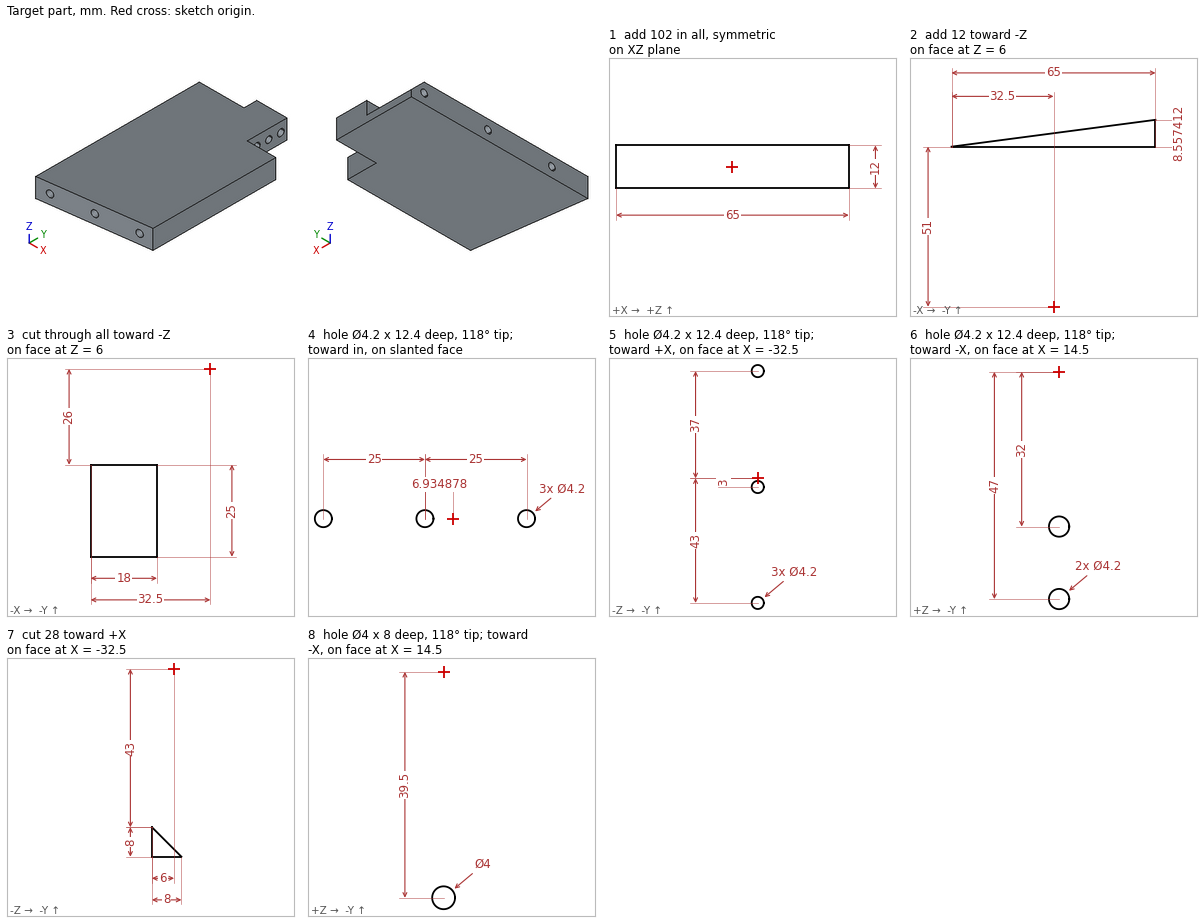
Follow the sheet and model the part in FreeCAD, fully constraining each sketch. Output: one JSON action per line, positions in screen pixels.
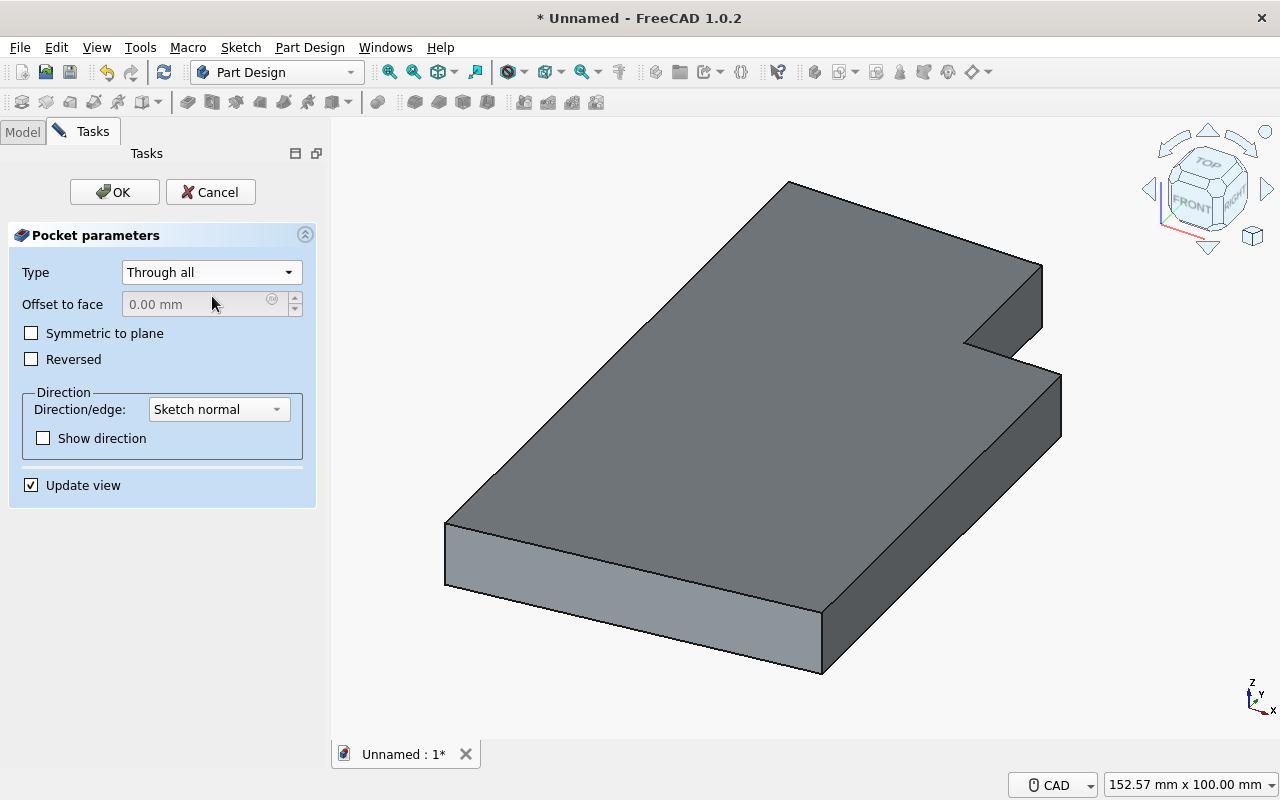
{"action": "left_click", "coordinate": [115, 192]}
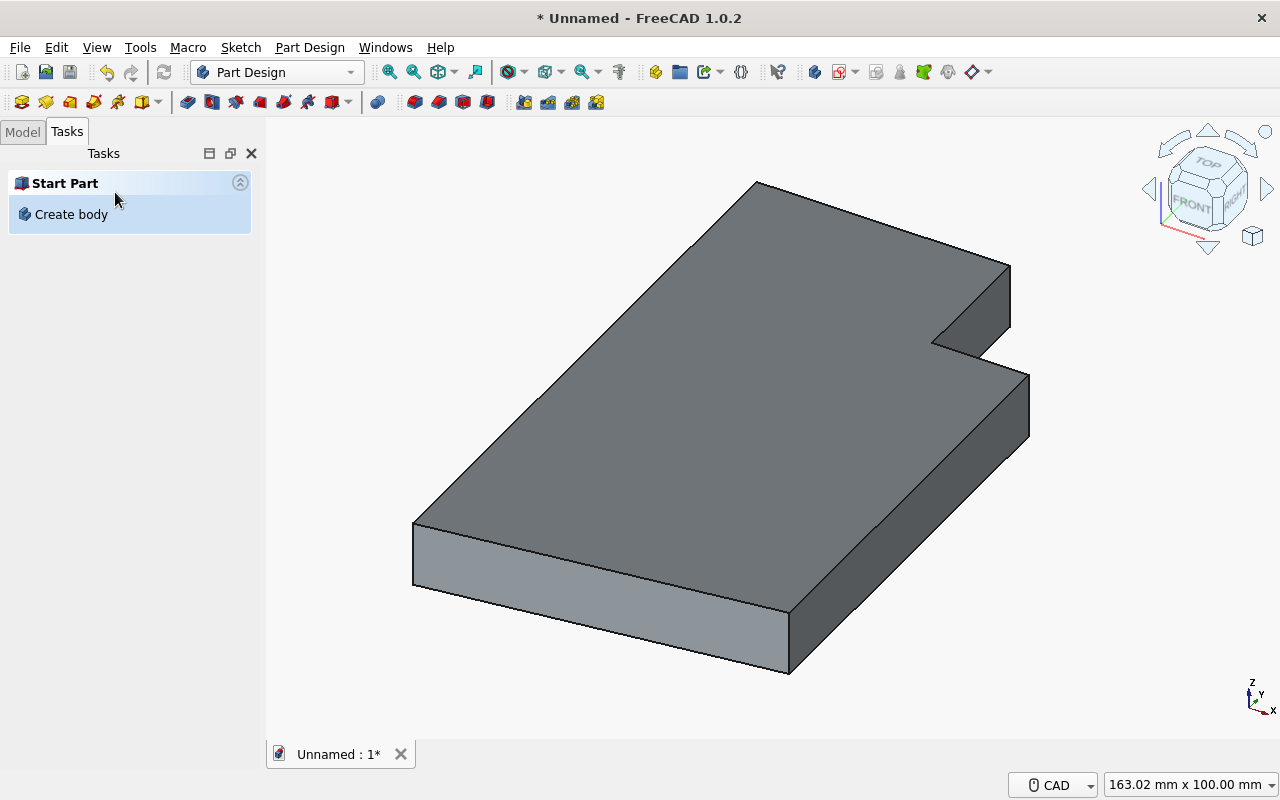
{"action": "left_click", "coordinate": [709, 623]}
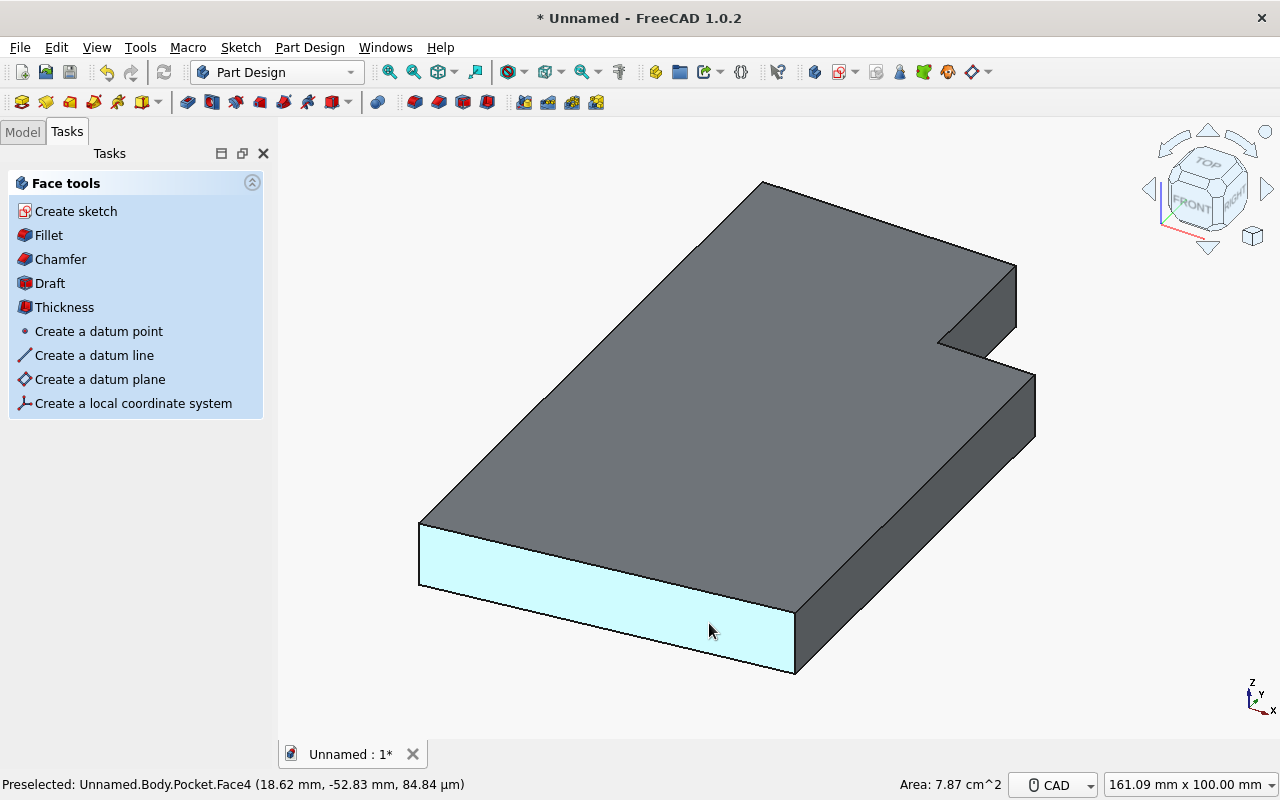
{"action": "left_click", "coordinate": [840, 72]}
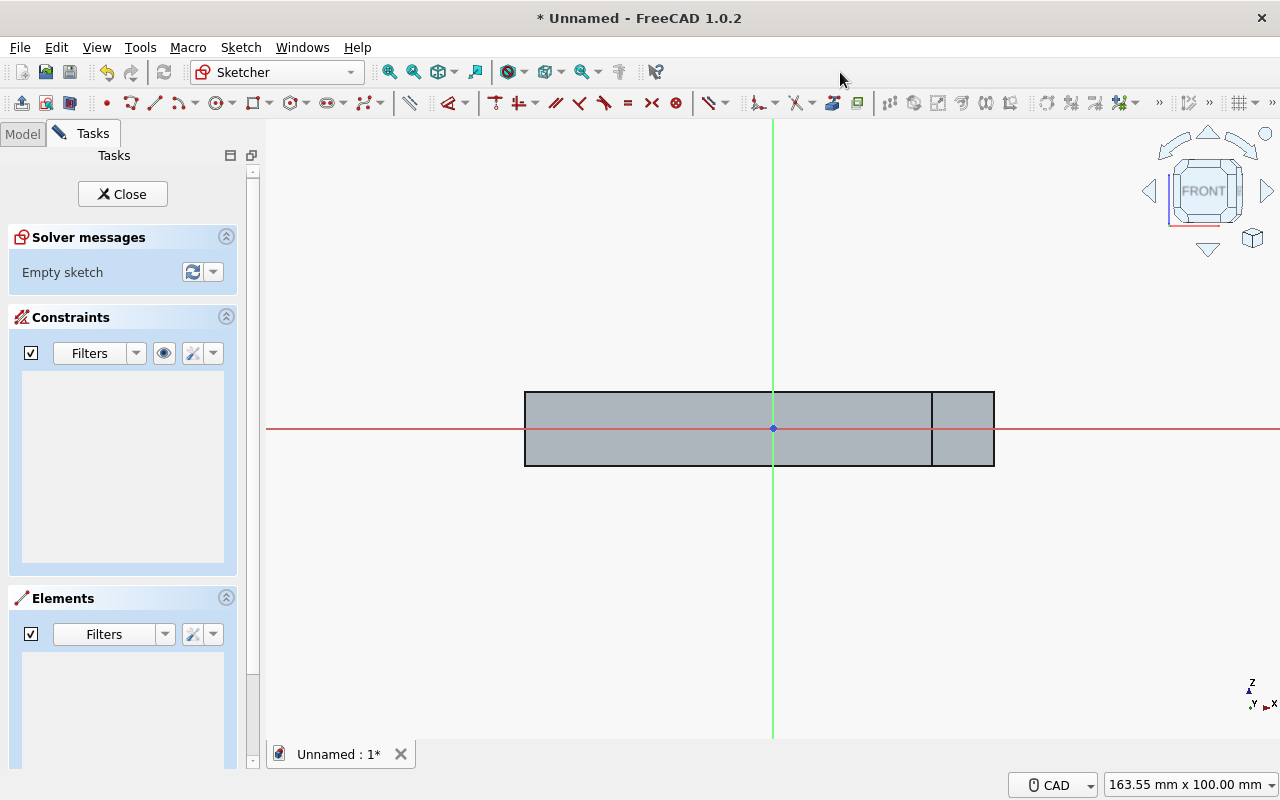
{"action": "key", "text": "q s"}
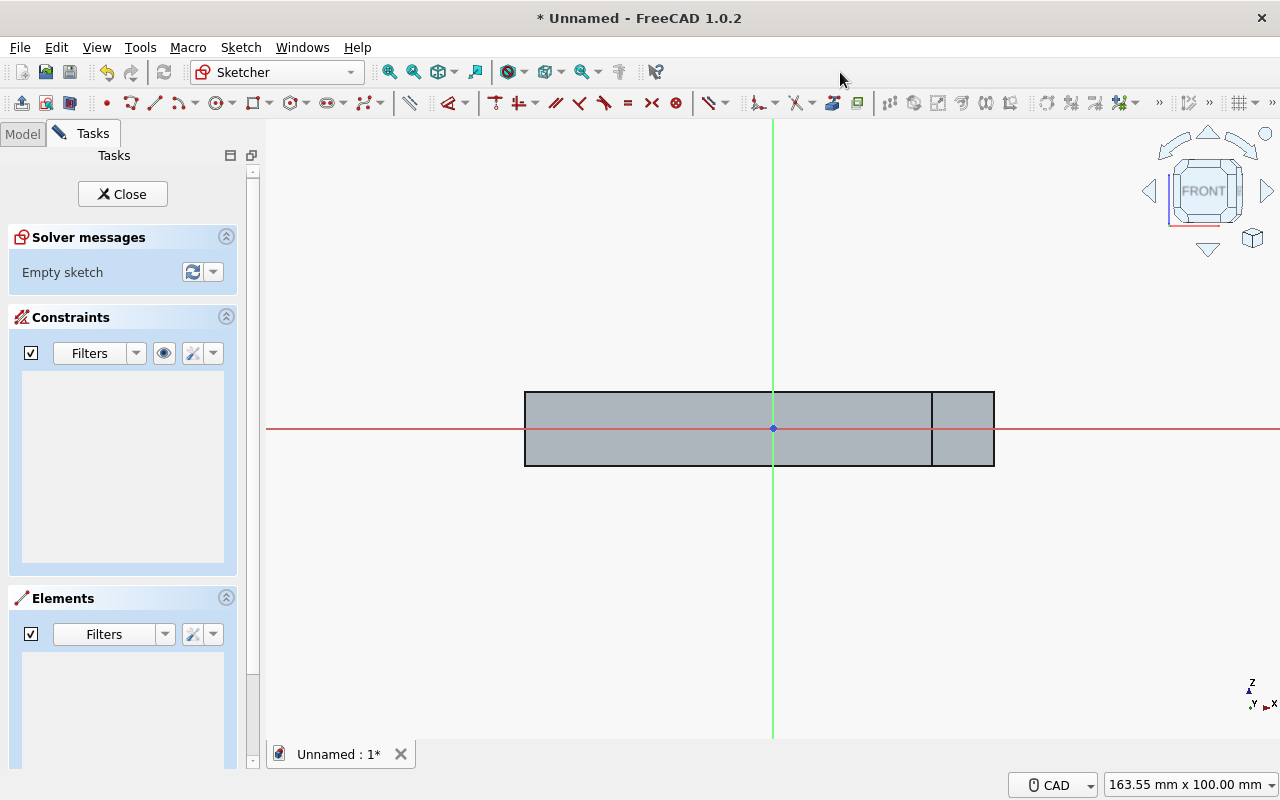
{"action": "scroll", "coordinate": [761, 429], "scroll_direction": "up", "scroll_amount": 3}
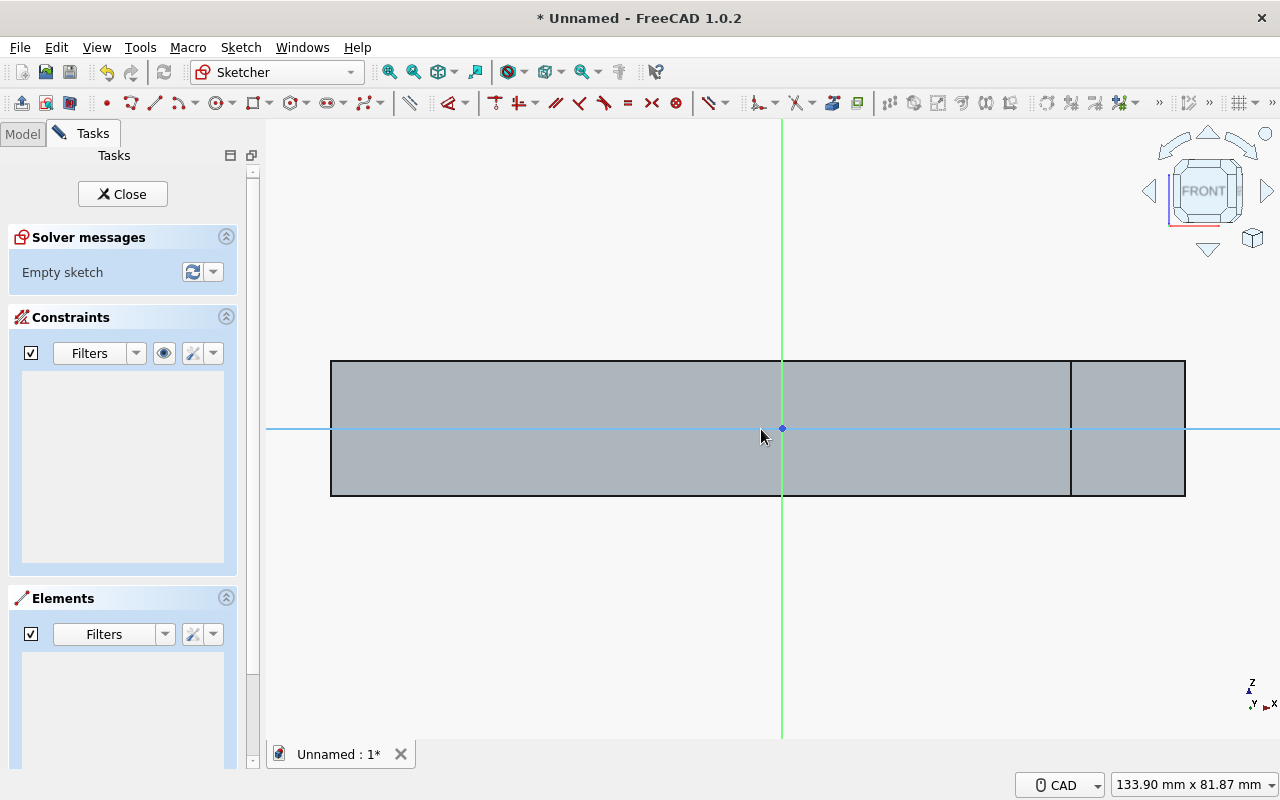
{"action": "left_click", "coordinate": [216, 104]}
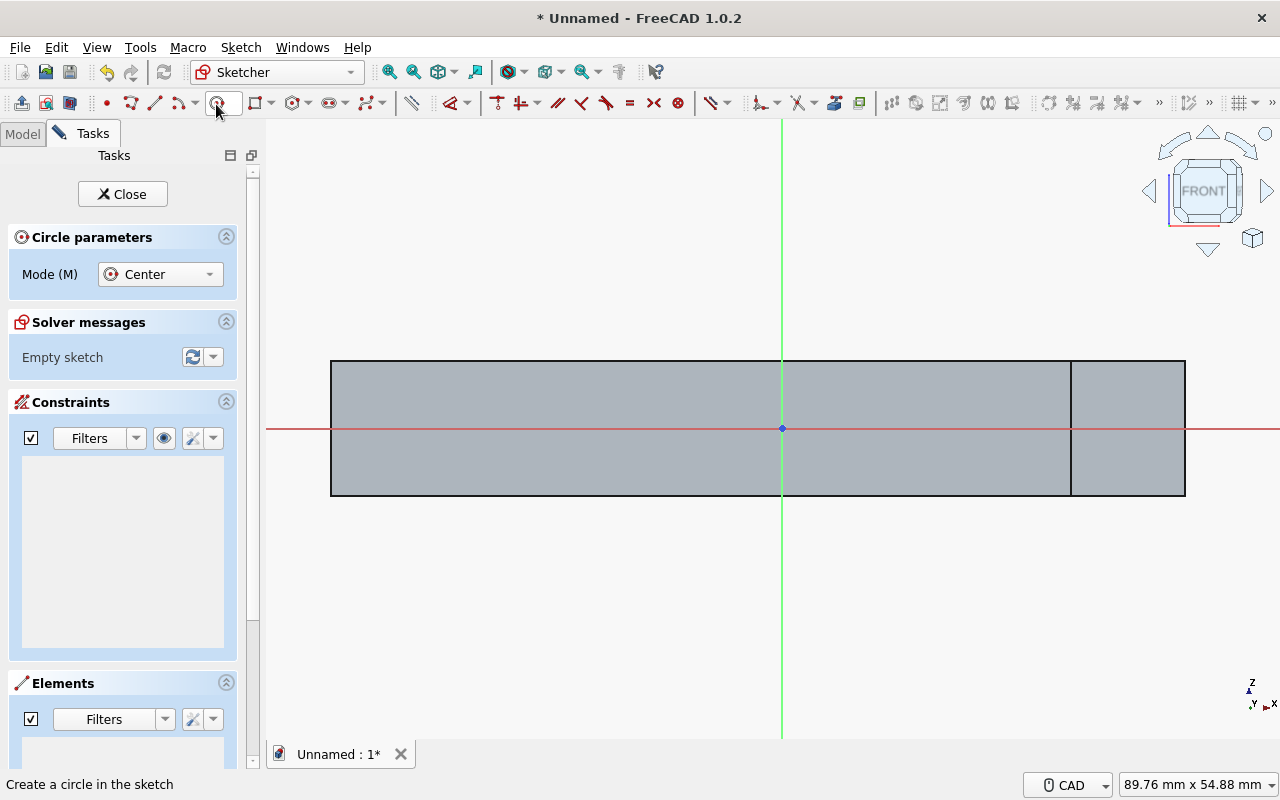
{"action": "left_click", "coordinate": [987, 429]}
{"action": "mouse_move", "coordinate": [1003, 412]}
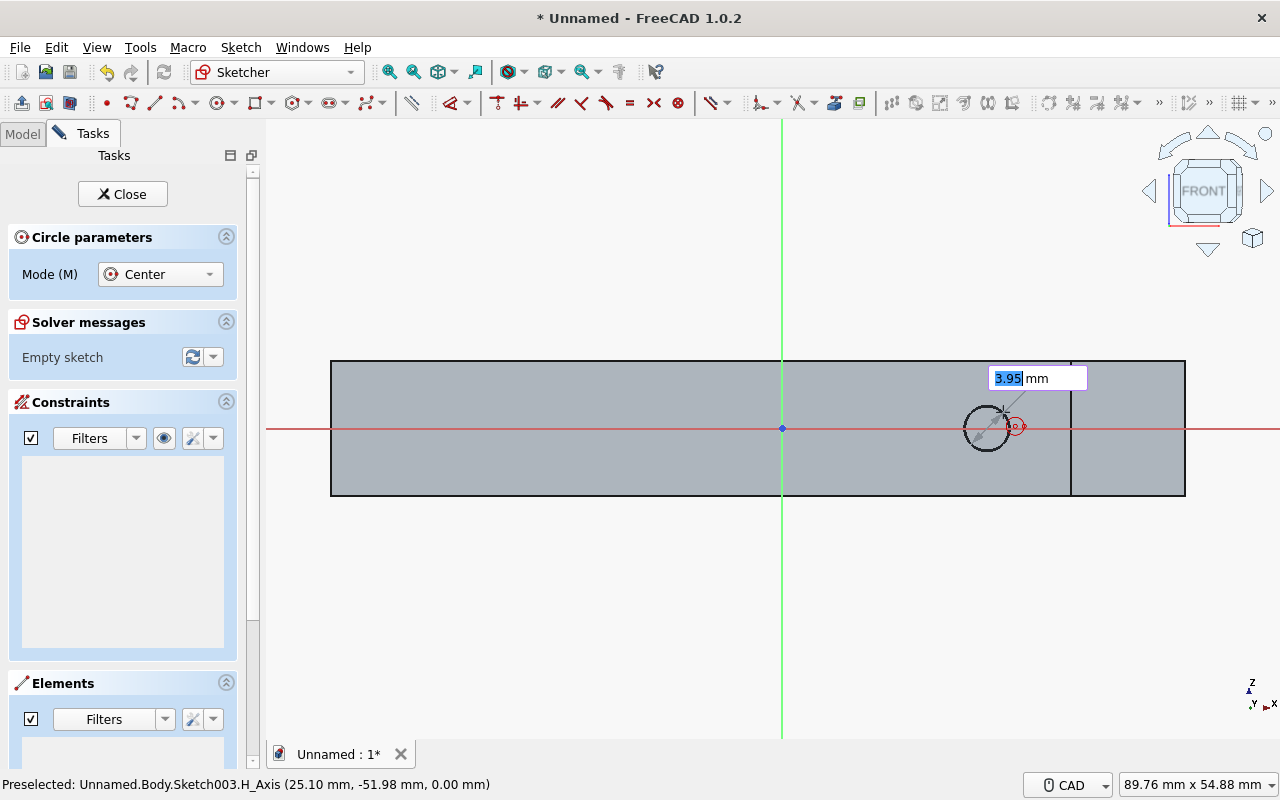
{"action": "type", "text": "4.2"}
{"action": "key", "text": "Return"}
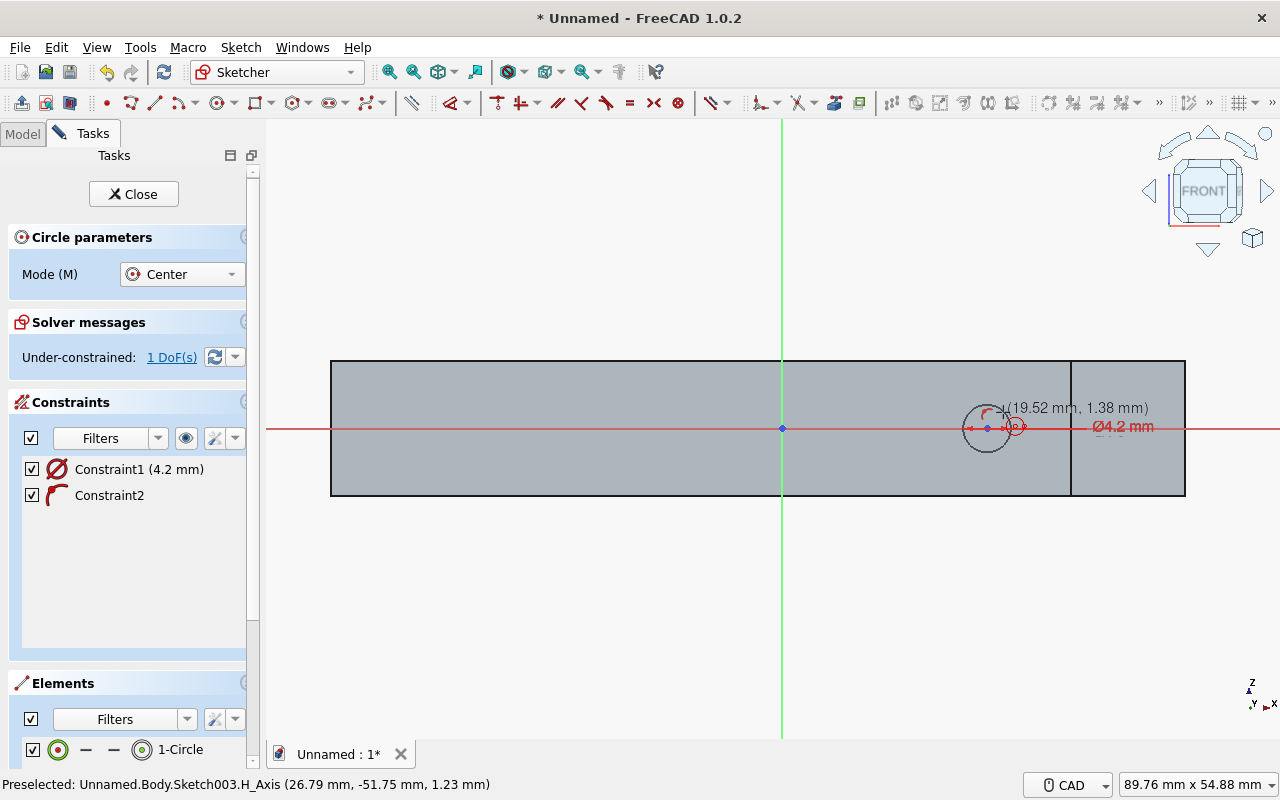
{"action": "left_click", "coordinate": [704, 429]}
{"action": "mouse_move", "coordinate": [721, 412]}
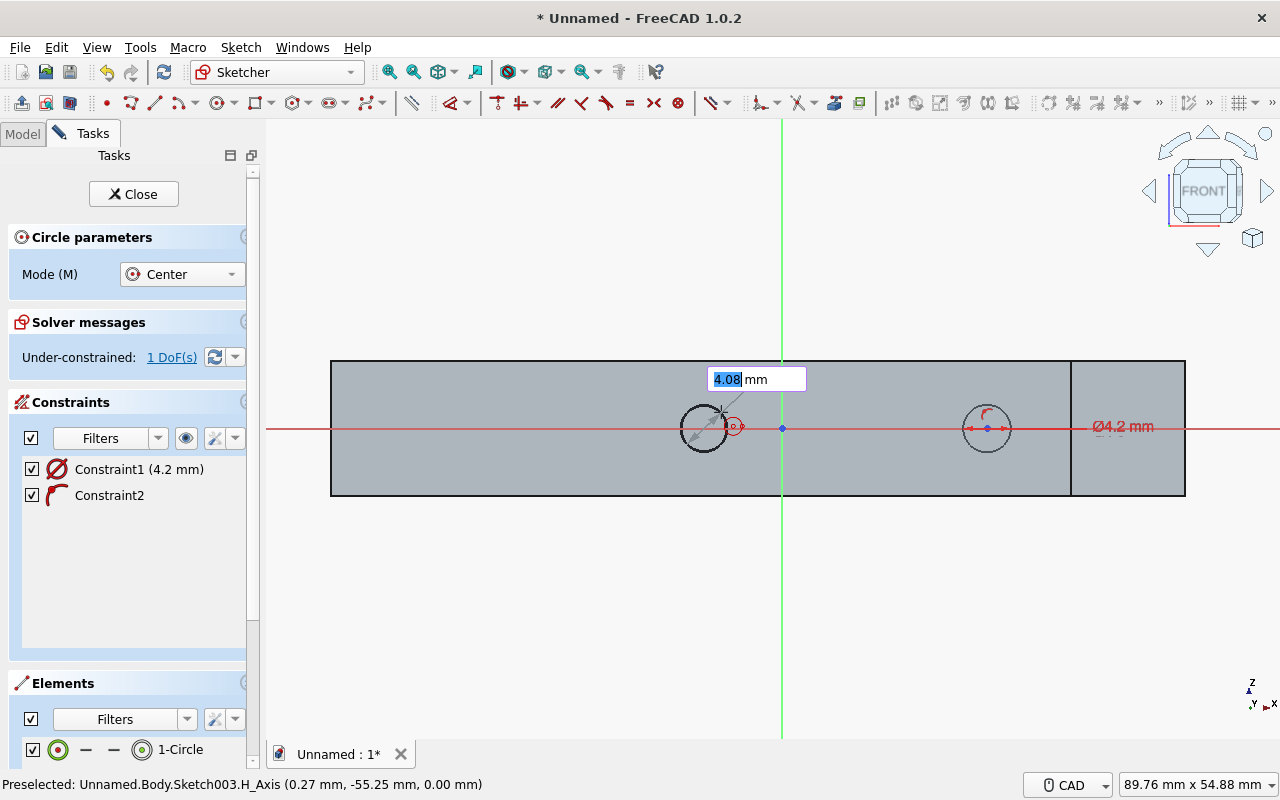
{"action": "type", "text": "4.2"}
{"action": "key", "text": "Return"}